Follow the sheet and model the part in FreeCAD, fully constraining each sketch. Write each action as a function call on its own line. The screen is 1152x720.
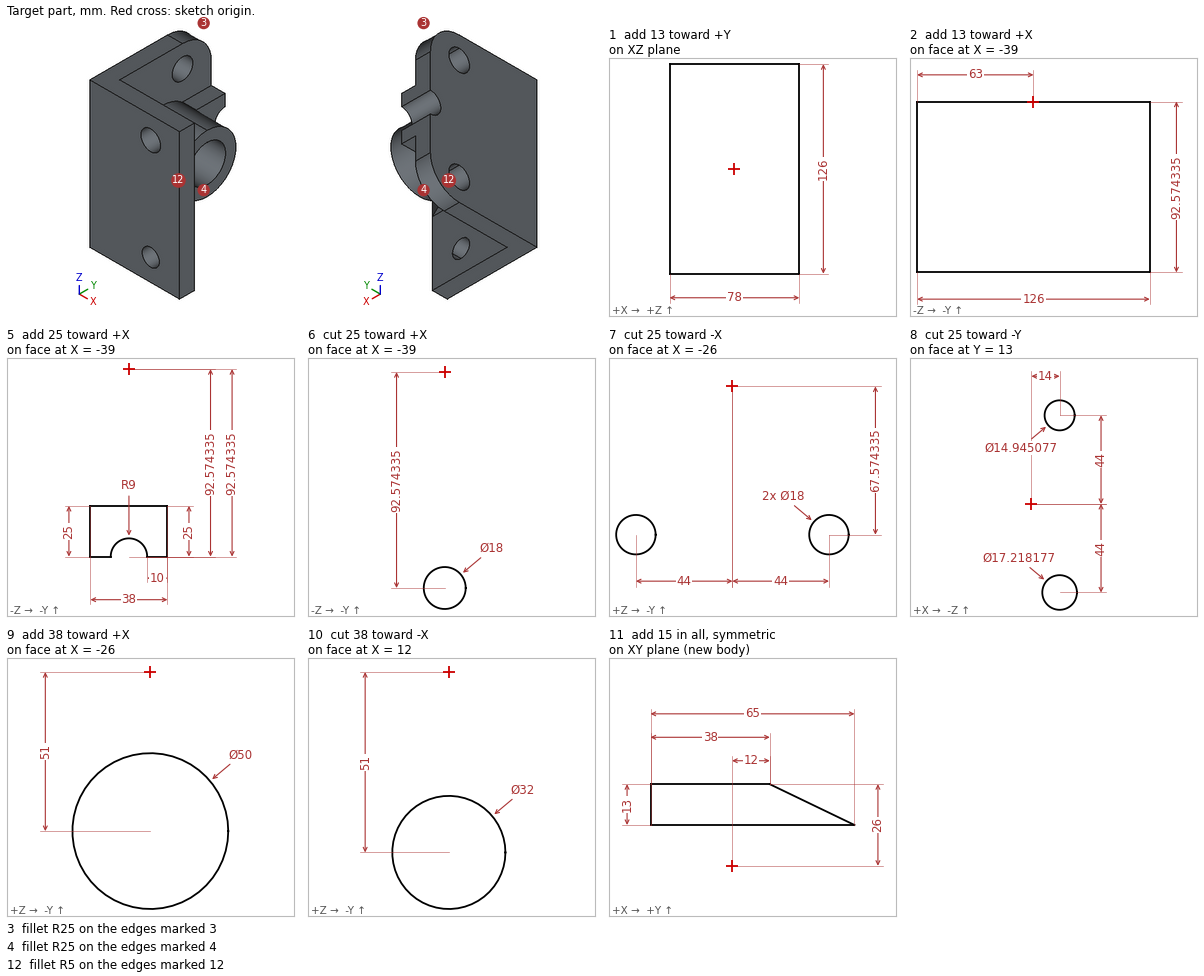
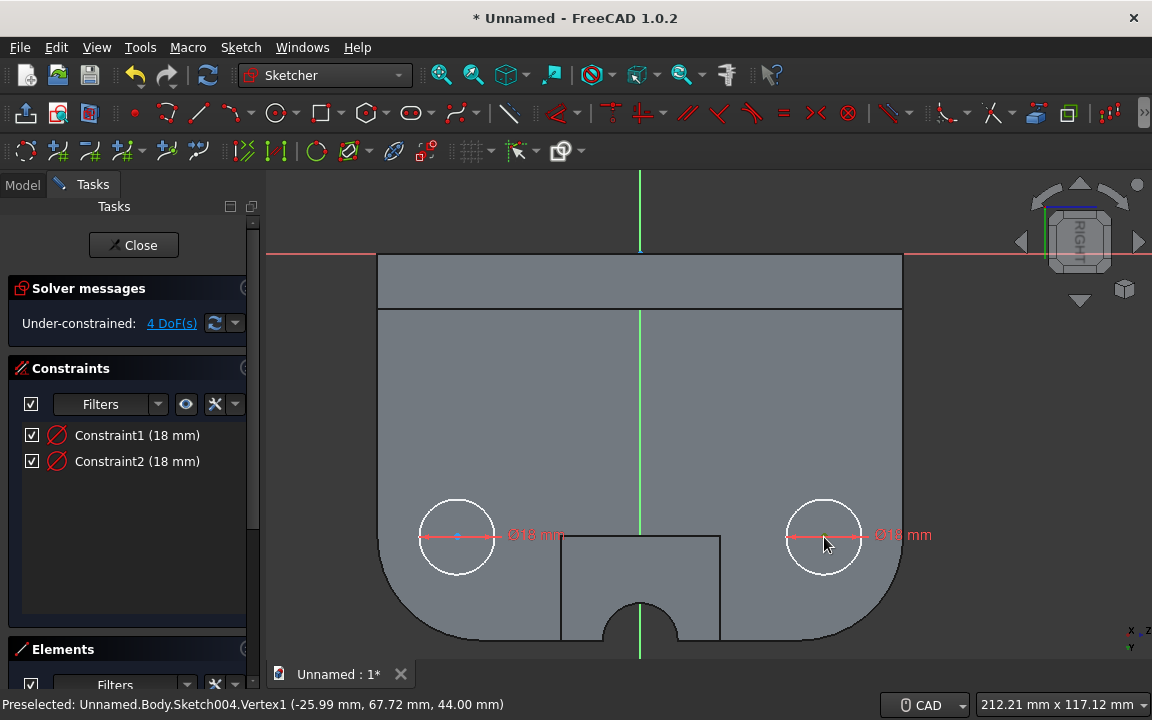
click(457, 537)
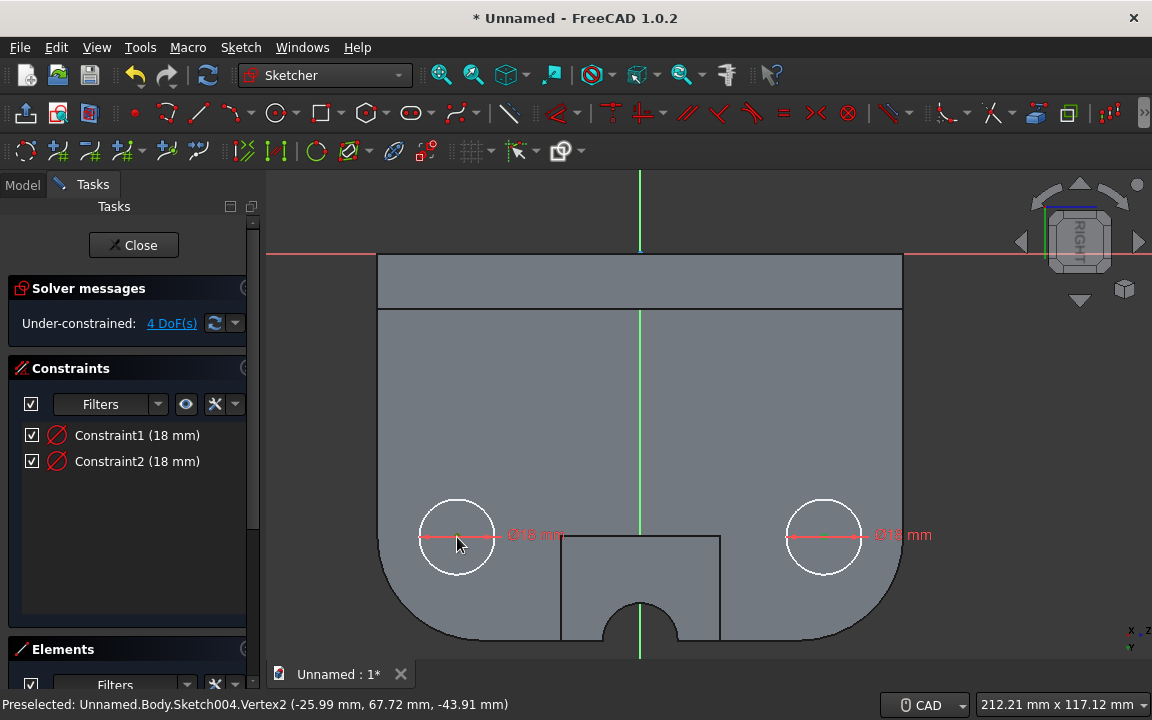
key(h)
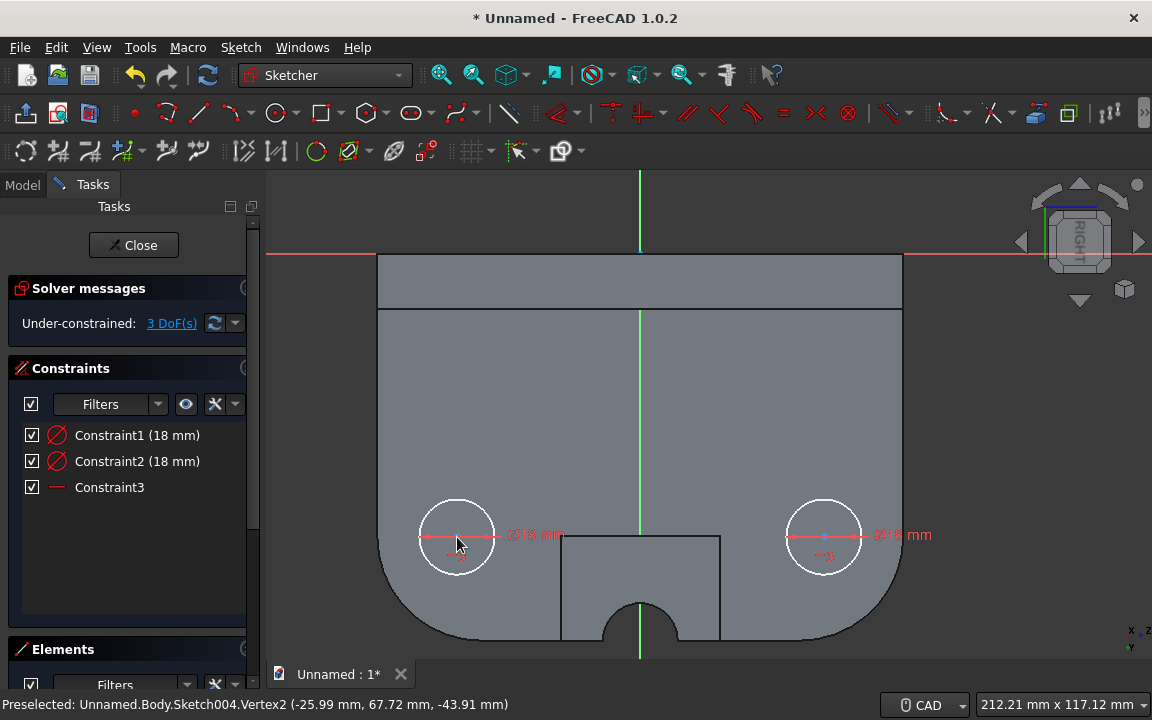
click(824, 537)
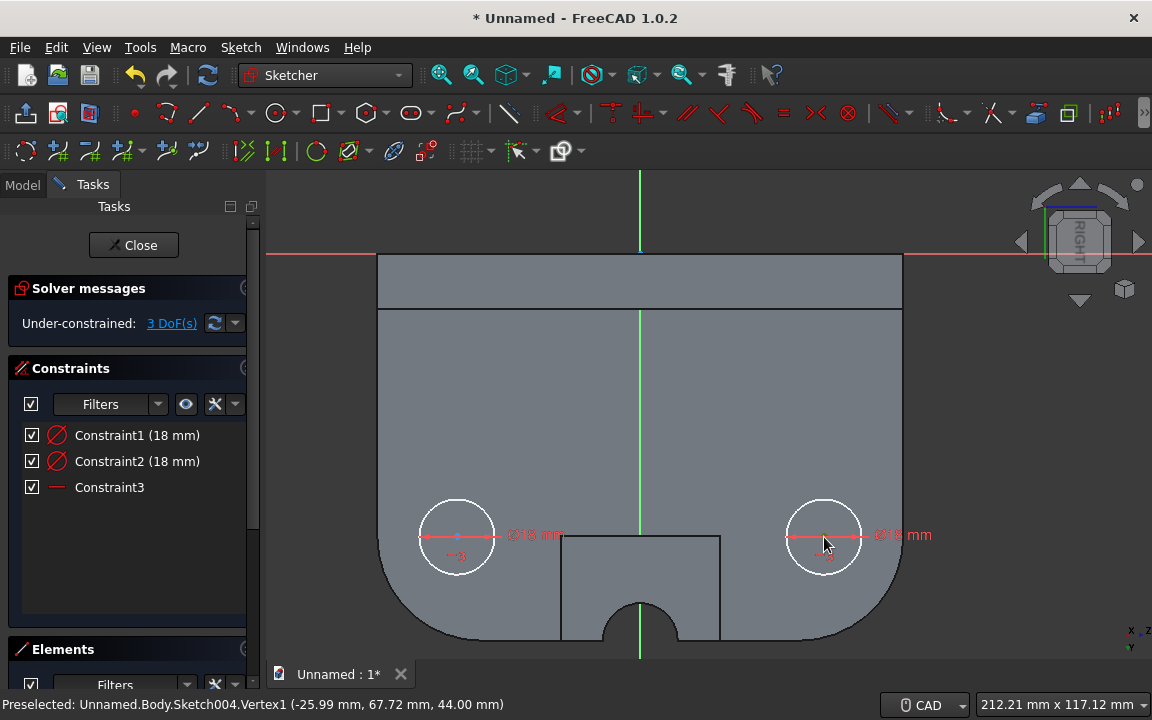
key(l)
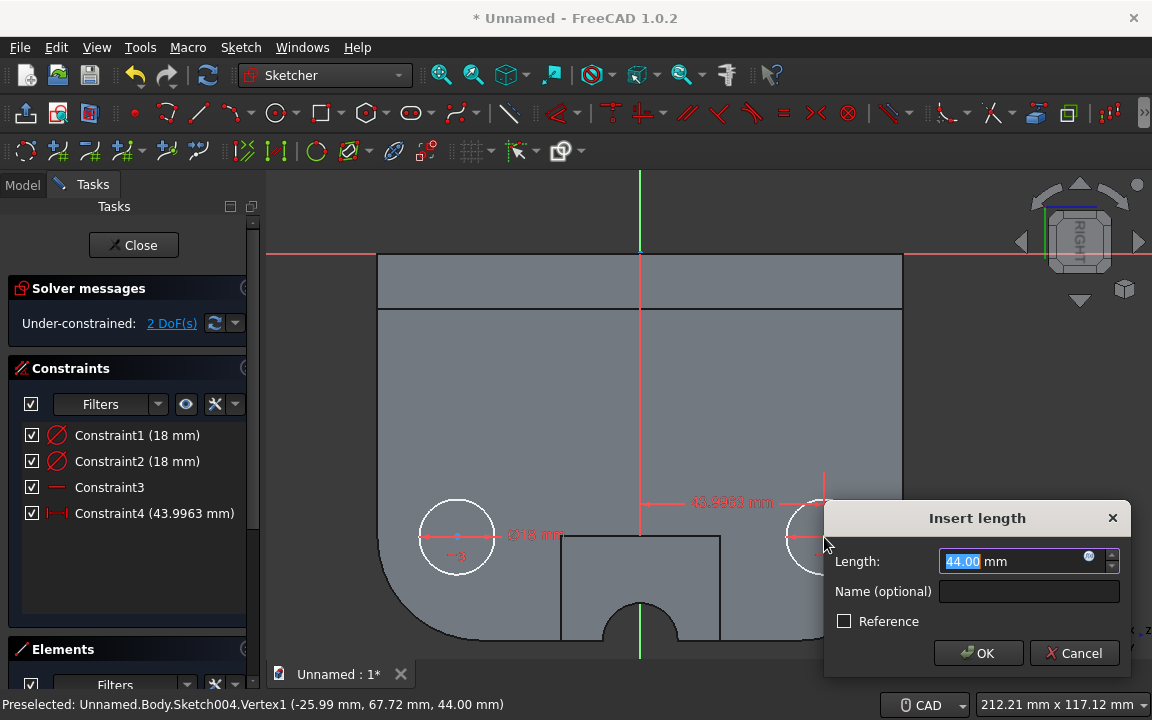
text(44)
key(Return)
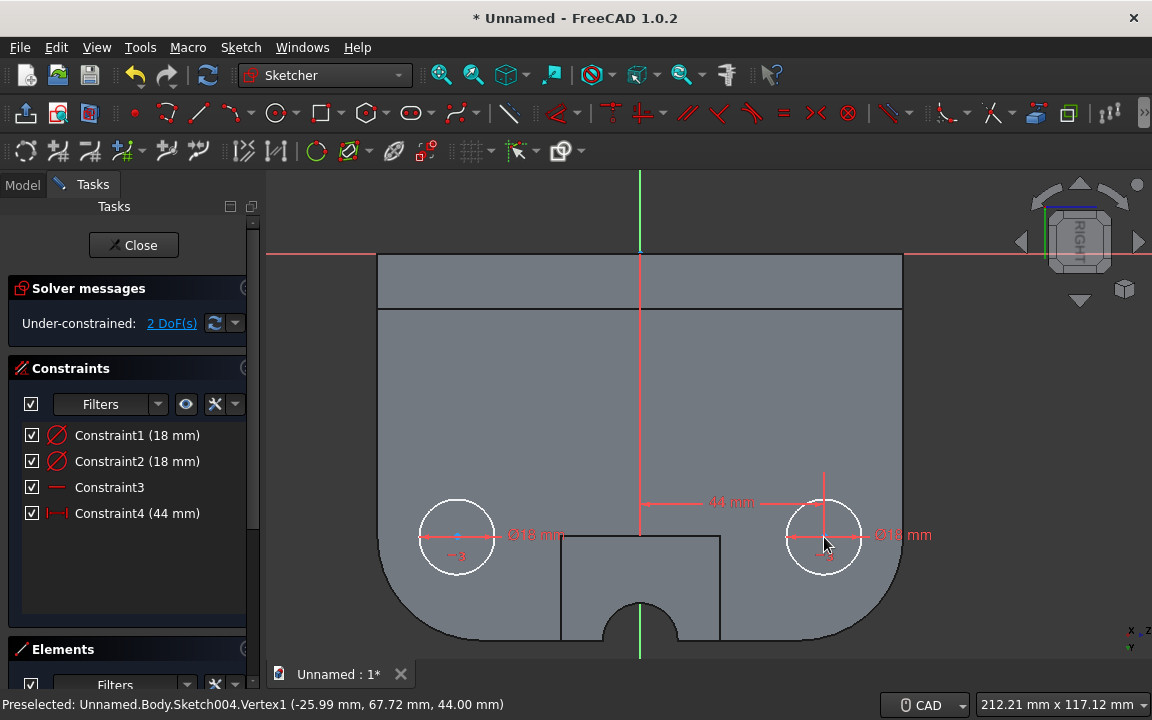
click(457, 537)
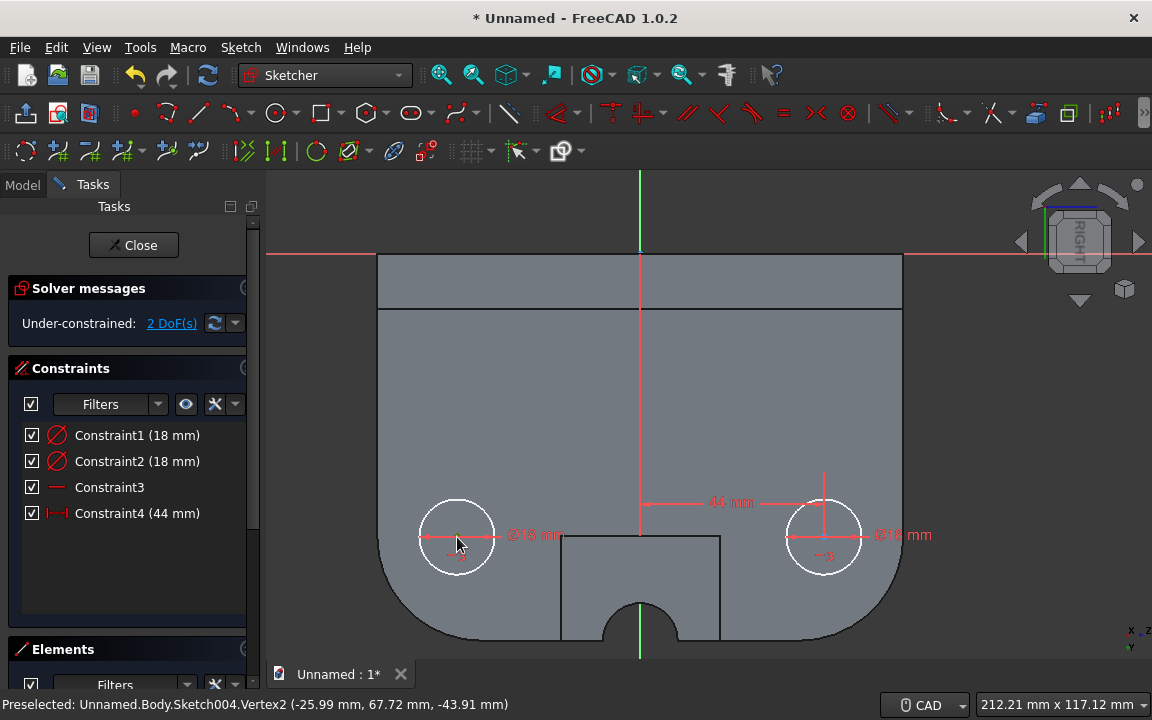
click(580, 114)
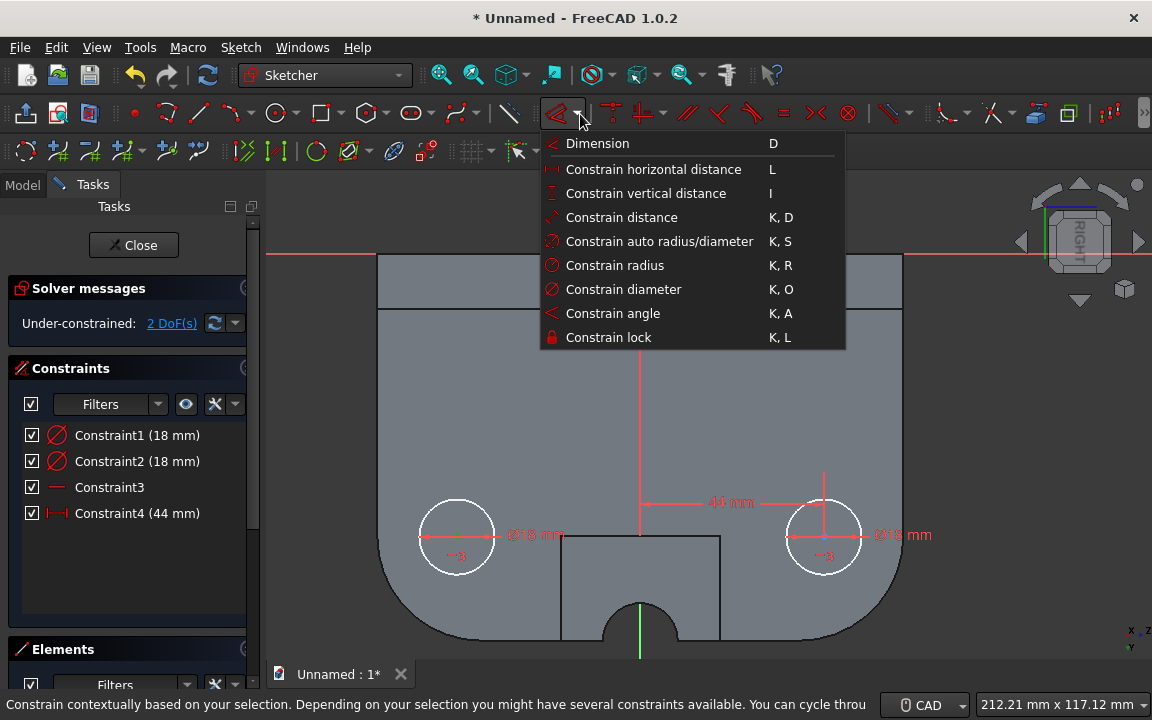
click(693, 169)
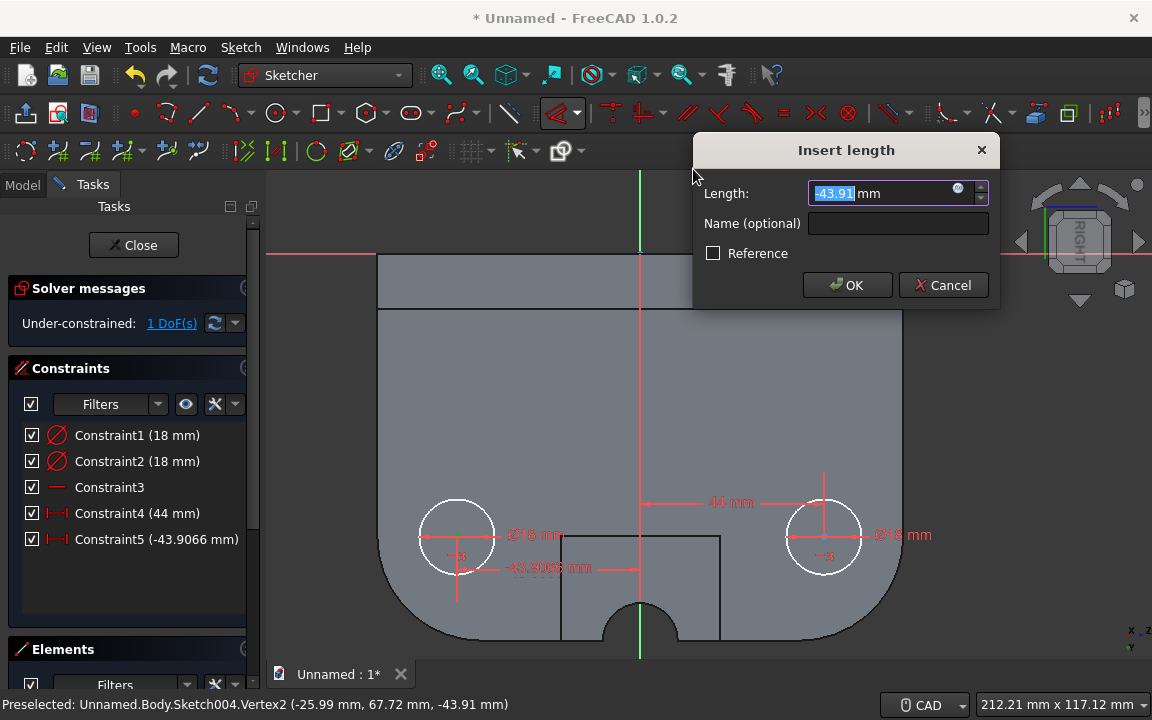
text(-44)
key(Return)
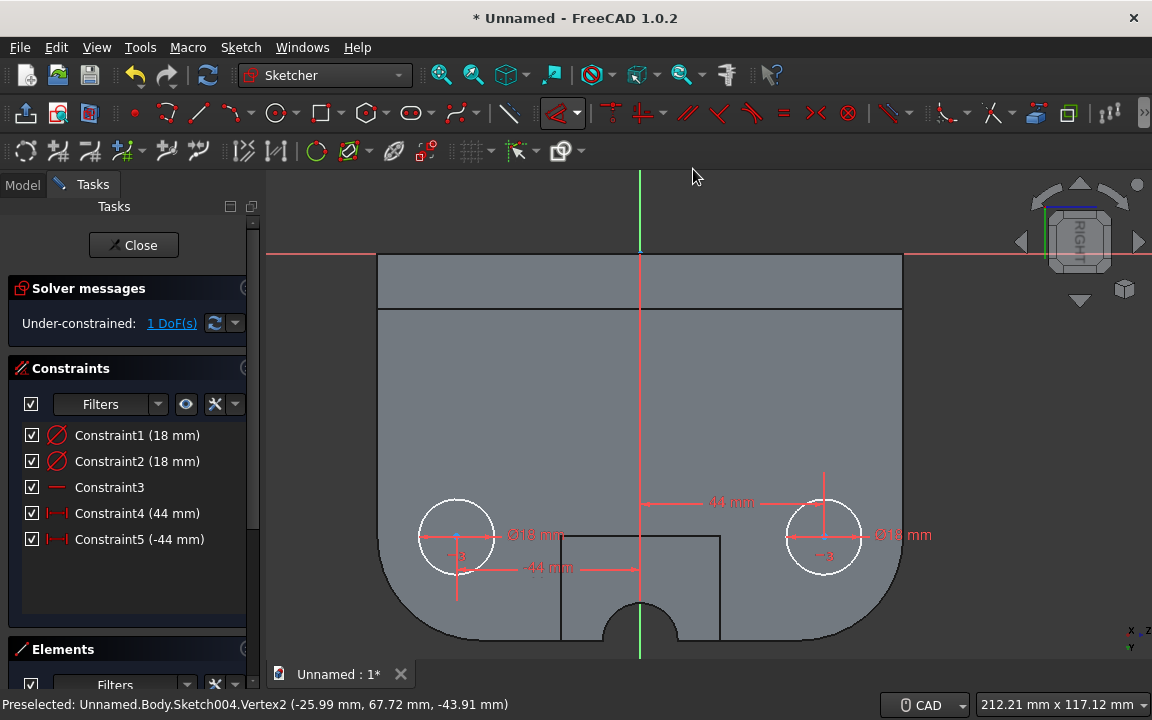
click(824, 537)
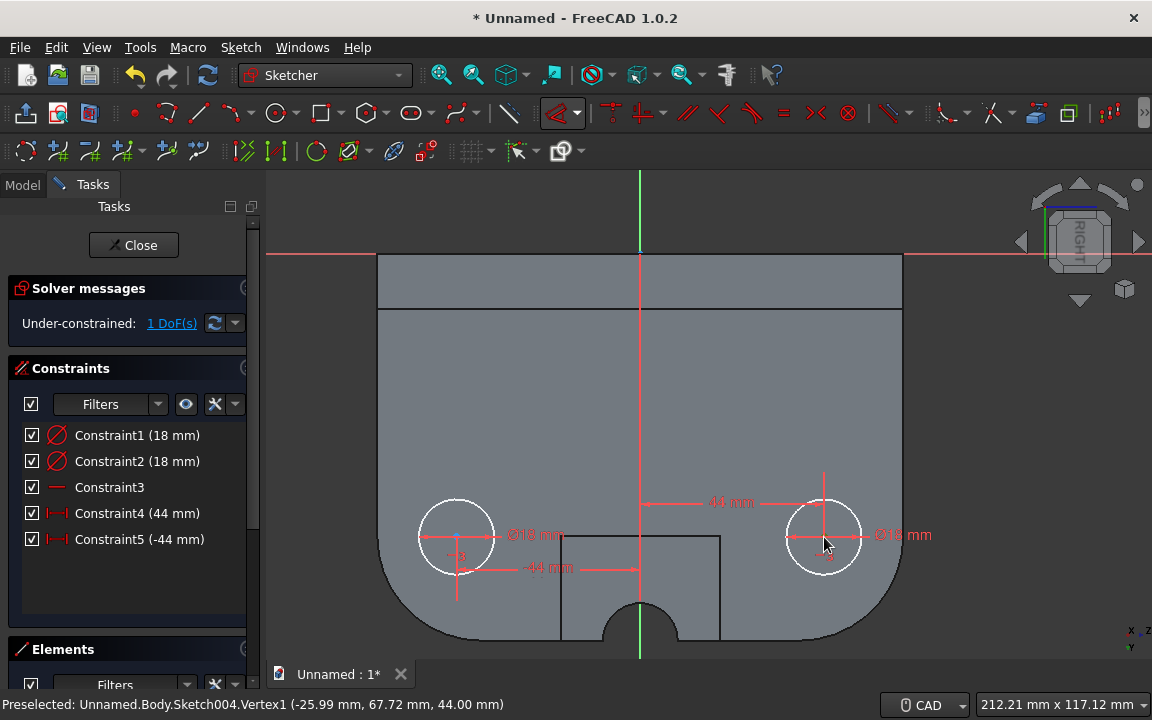
key(i)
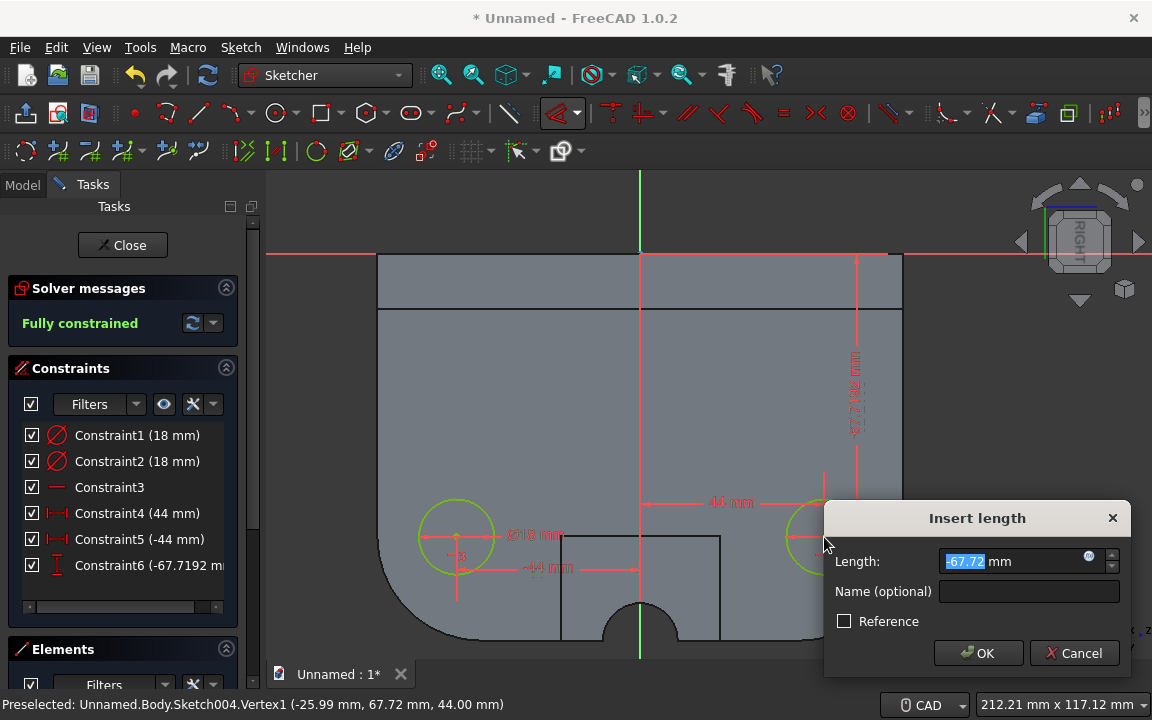
text(-67.574335)
key(Return)